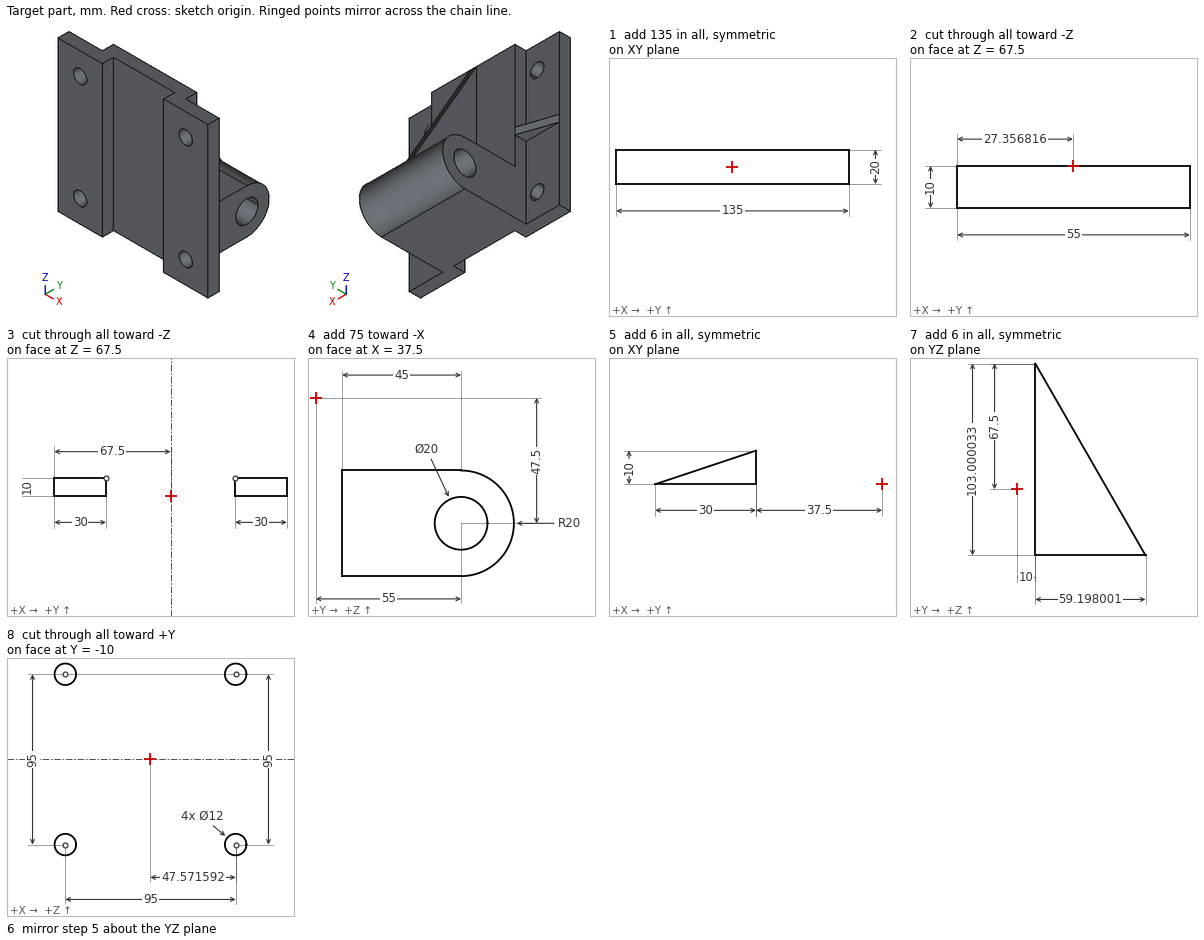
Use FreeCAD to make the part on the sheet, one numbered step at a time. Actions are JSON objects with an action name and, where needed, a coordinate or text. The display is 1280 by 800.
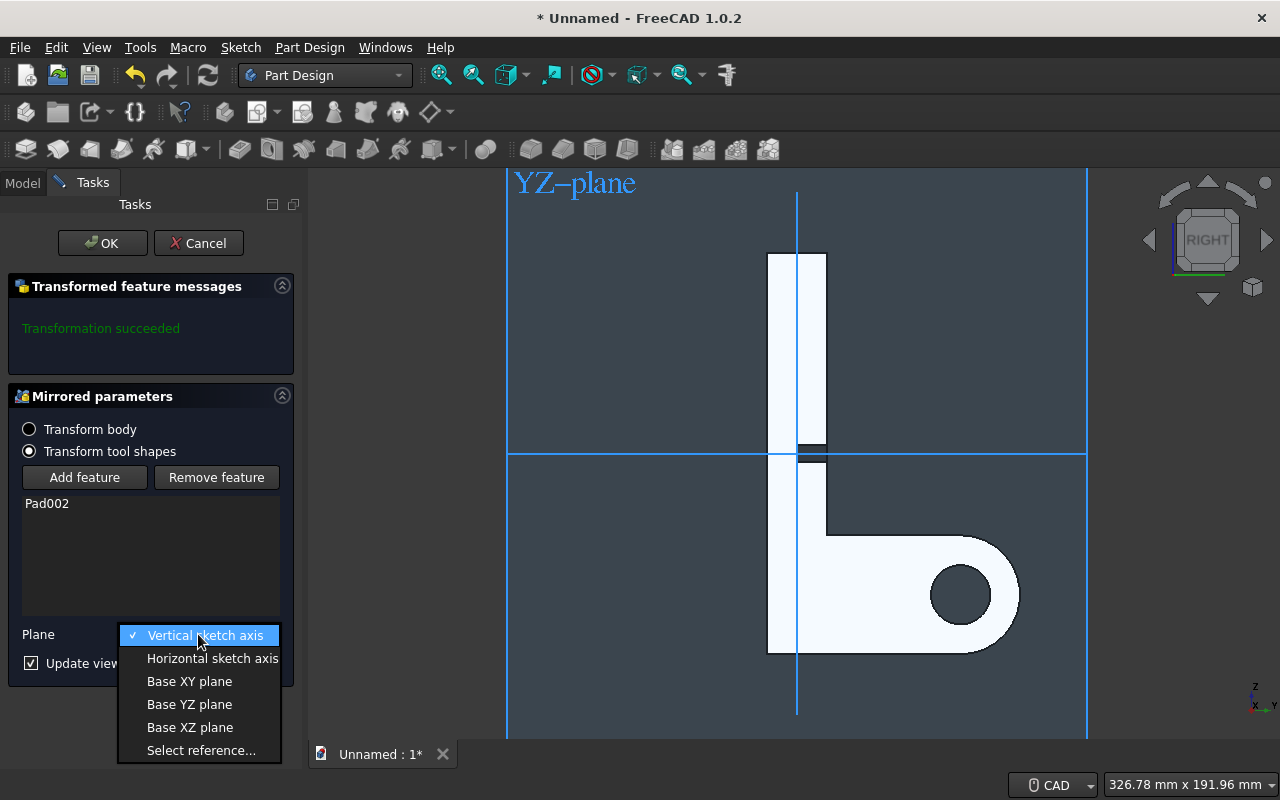
{"action": "left_click", "coordinate": [198, 704]}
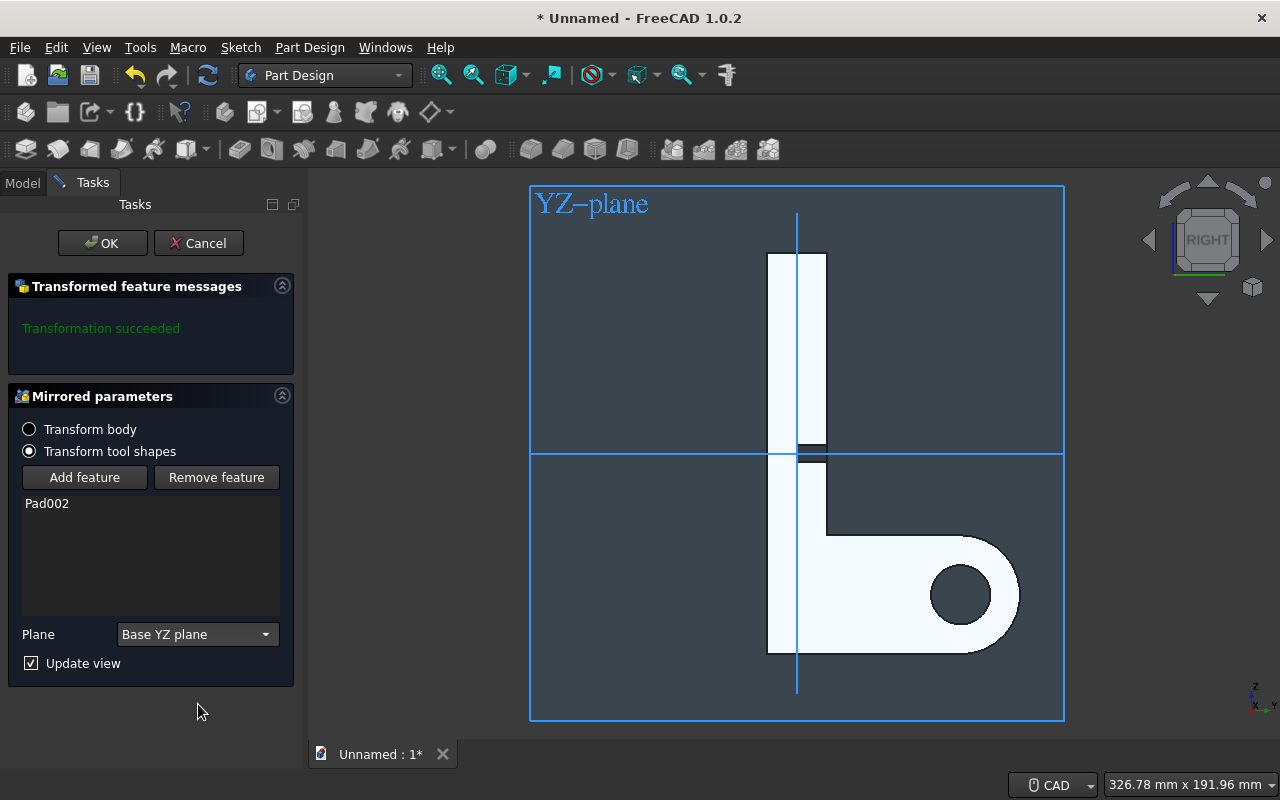
{"action": "left_click", "coordinate": [103, 243]}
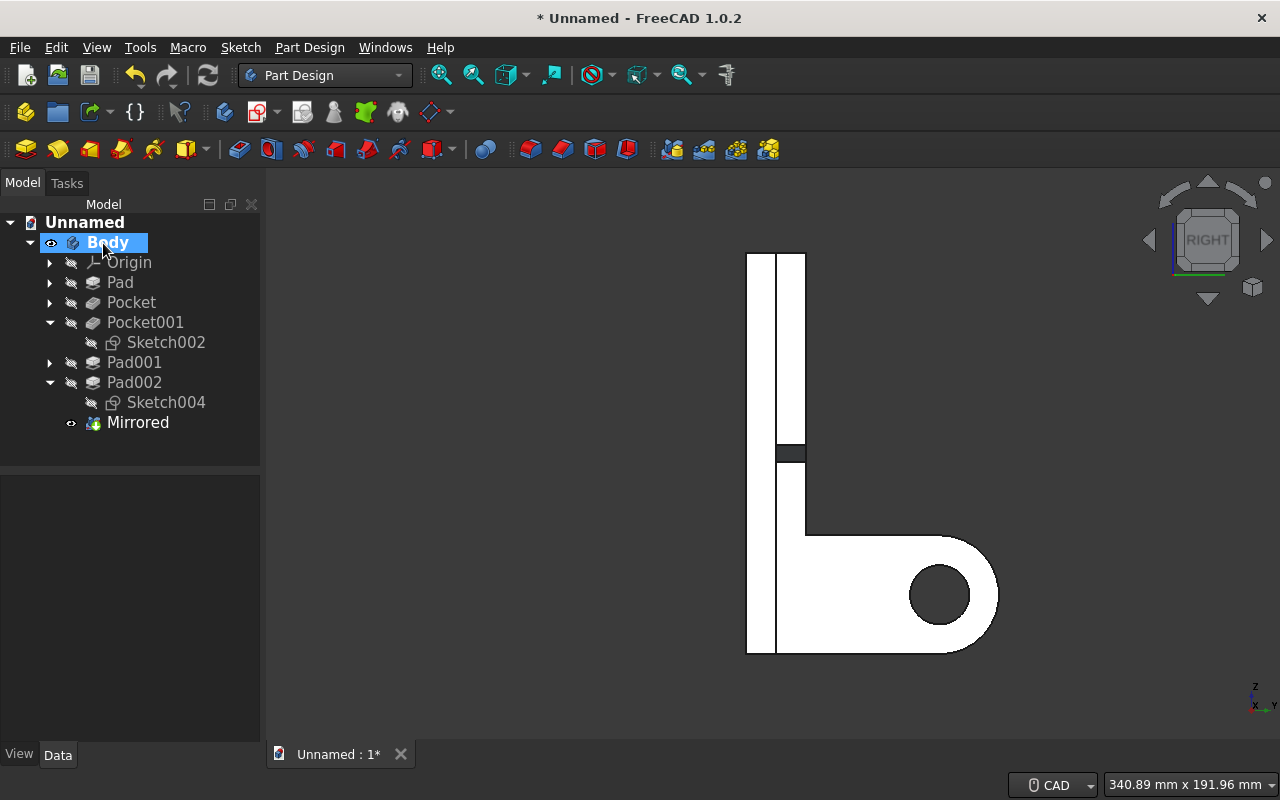
{"action": "left_click", "coordinate": [258, 112]}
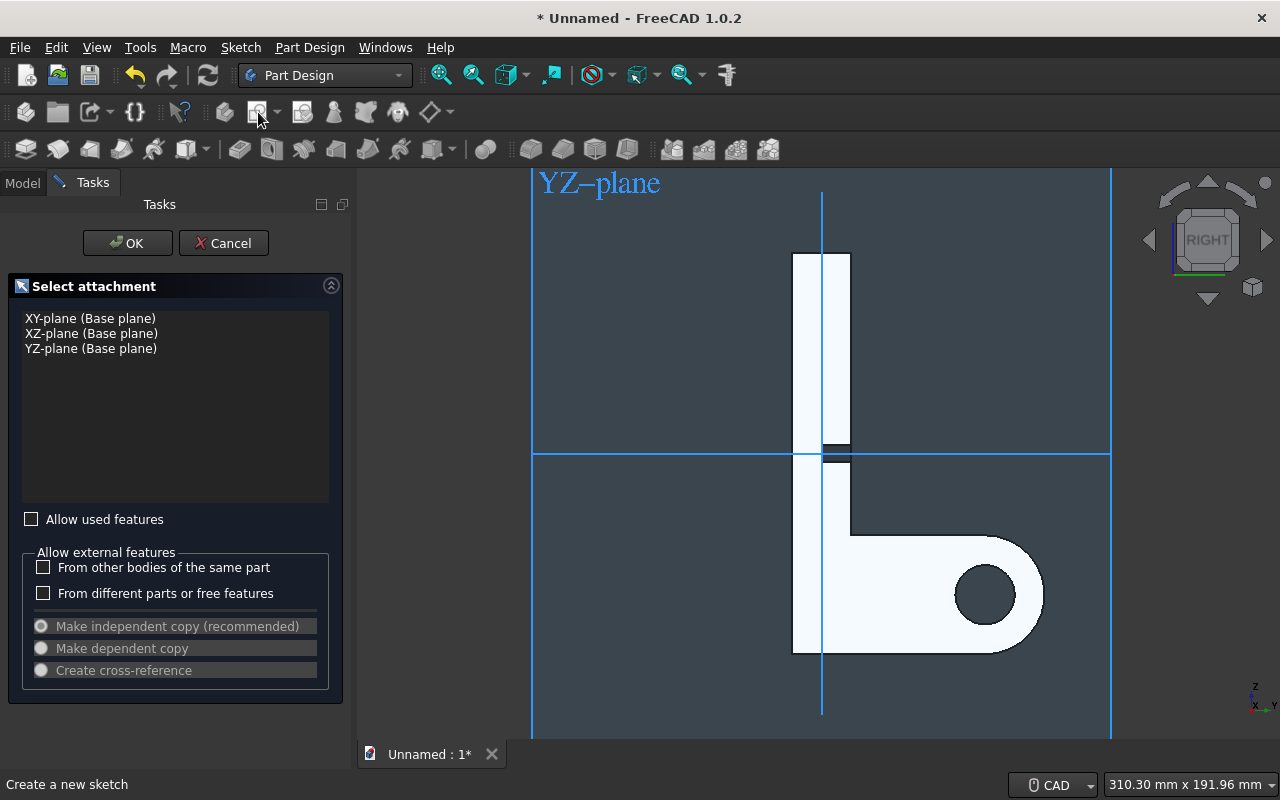
{"action": "left_click", "coordinate": [82, 348]}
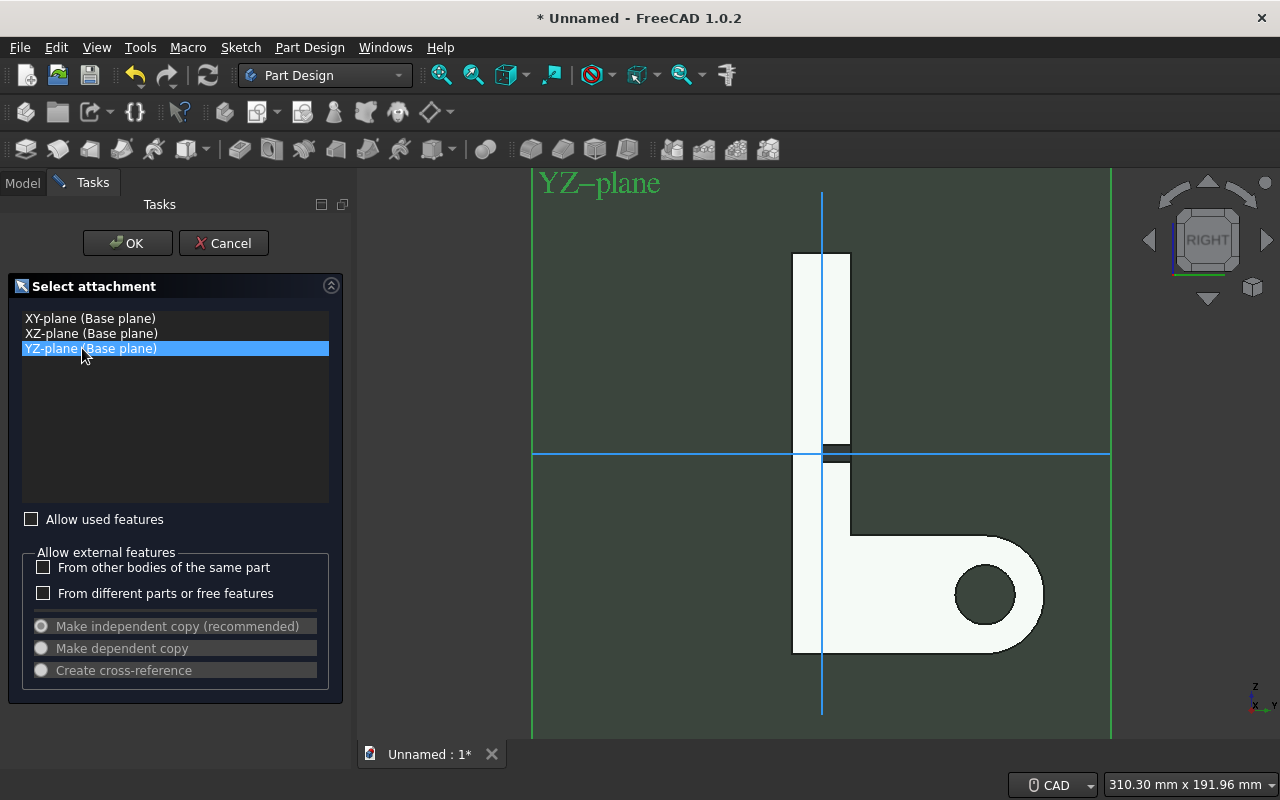
{"action": "left_click", "coordinate": [128, 243]}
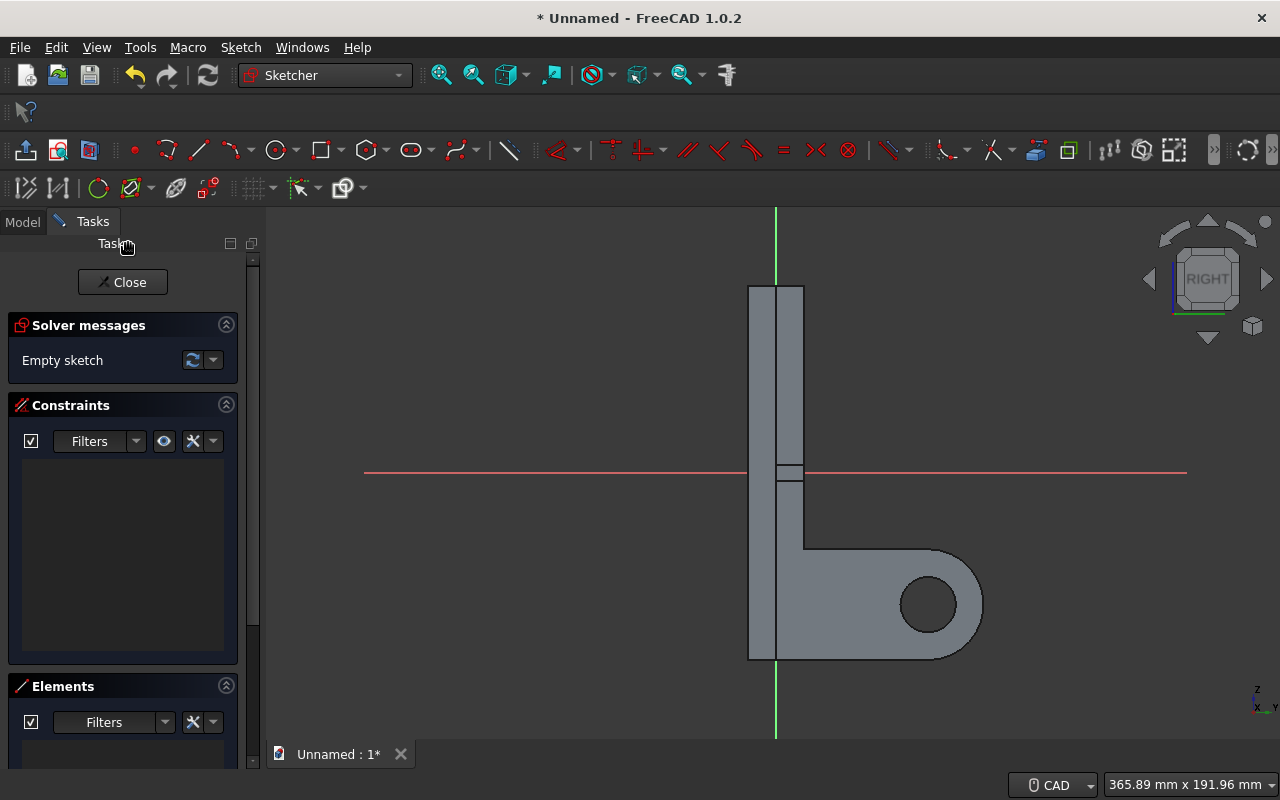
{"action": "key", "text": "q s"}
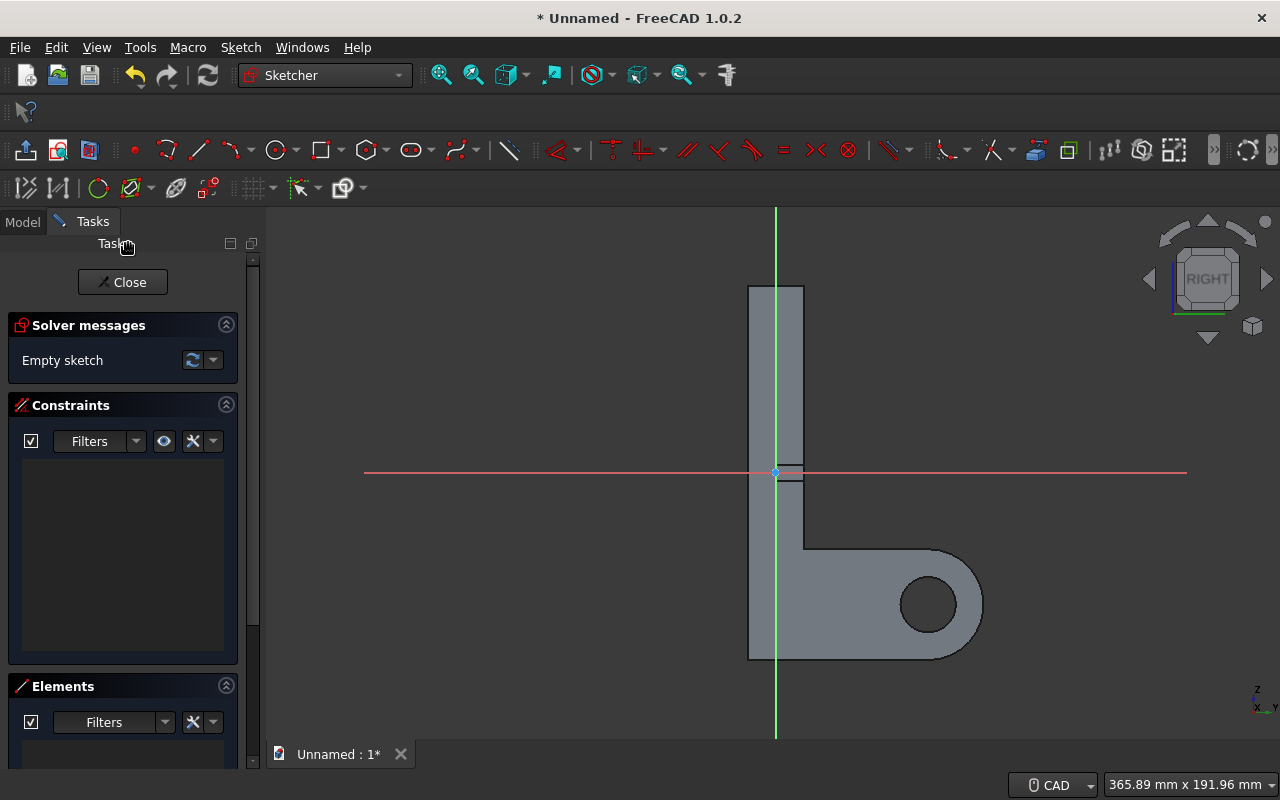
{"action": "key", "text": "g m"}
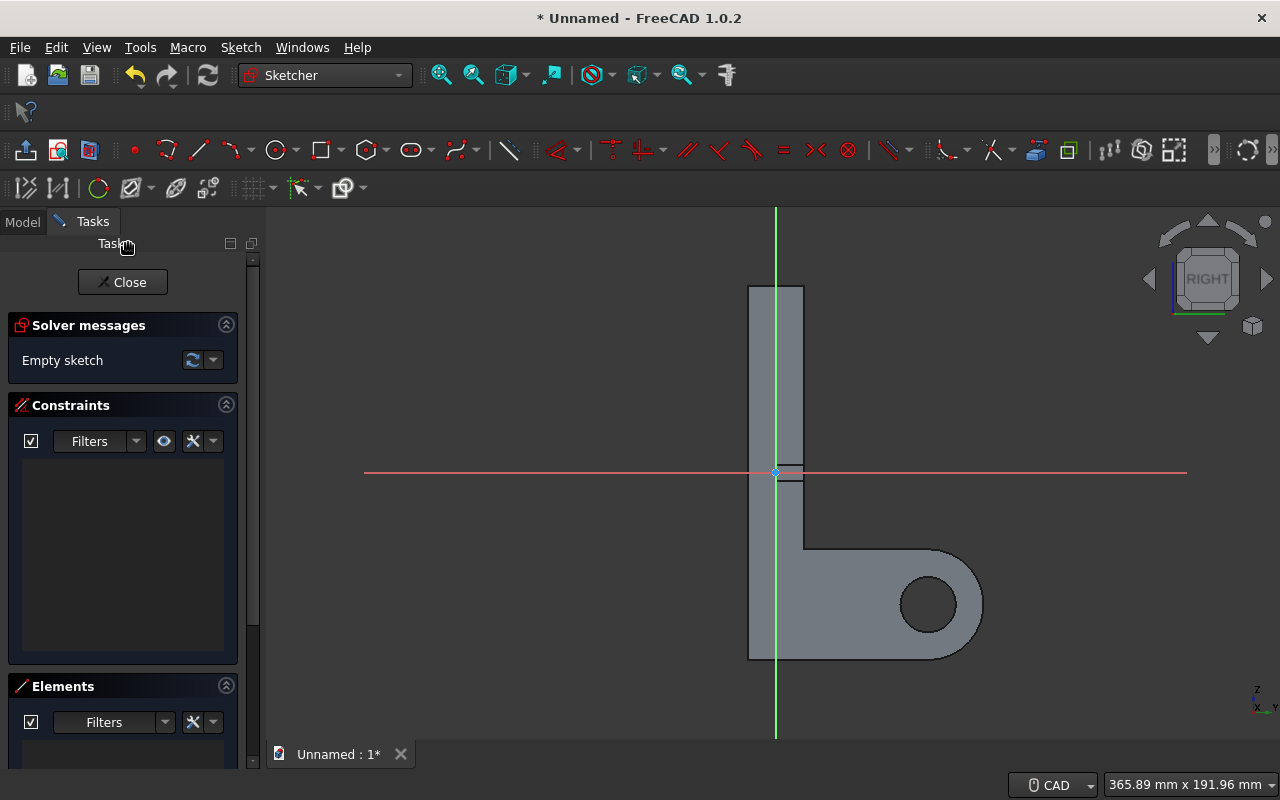
{"action": "left_click", "coordinate": [804, 571]}
{"action": "left_click", "coordinate": [968, 571]}
{"action": "left_click", "coordinate": [804, 286]}
{"action": "left_click", "coordinate": [804, 572]}
{"action": "key", "text": "Escape"}
{"action": "key", "text": "Escape"}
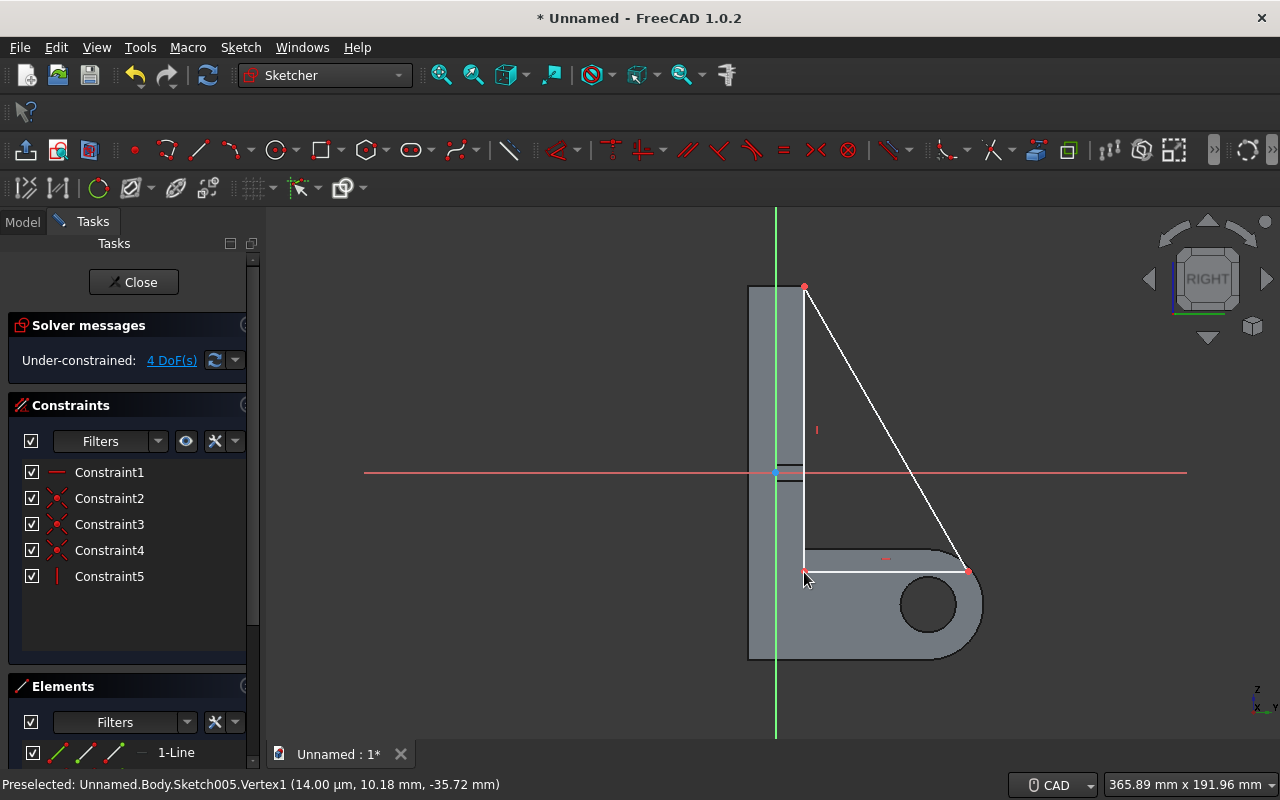
{"action": "left_click", "coordinate": [556, 150]}